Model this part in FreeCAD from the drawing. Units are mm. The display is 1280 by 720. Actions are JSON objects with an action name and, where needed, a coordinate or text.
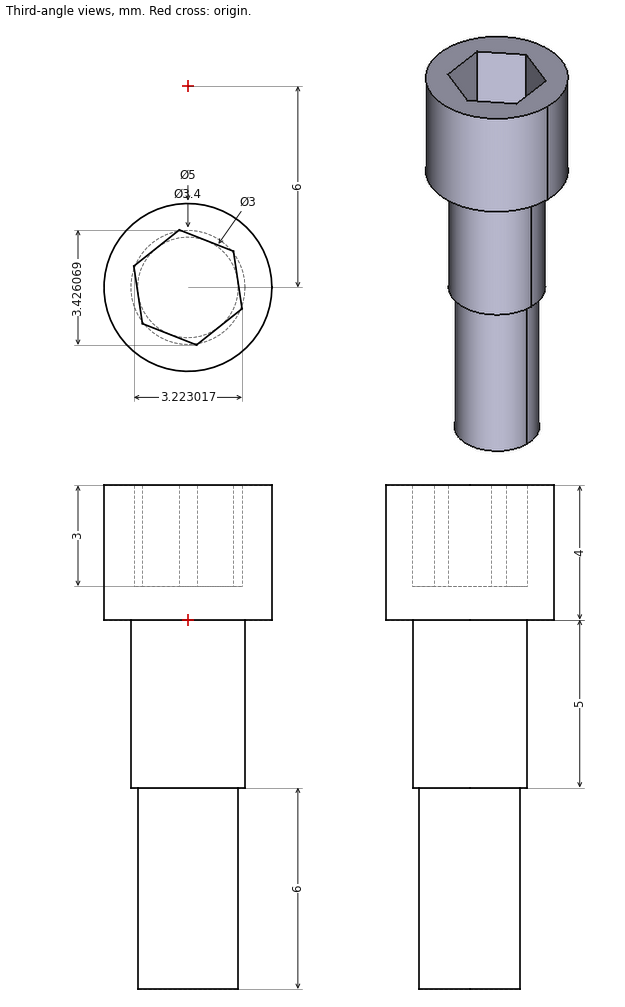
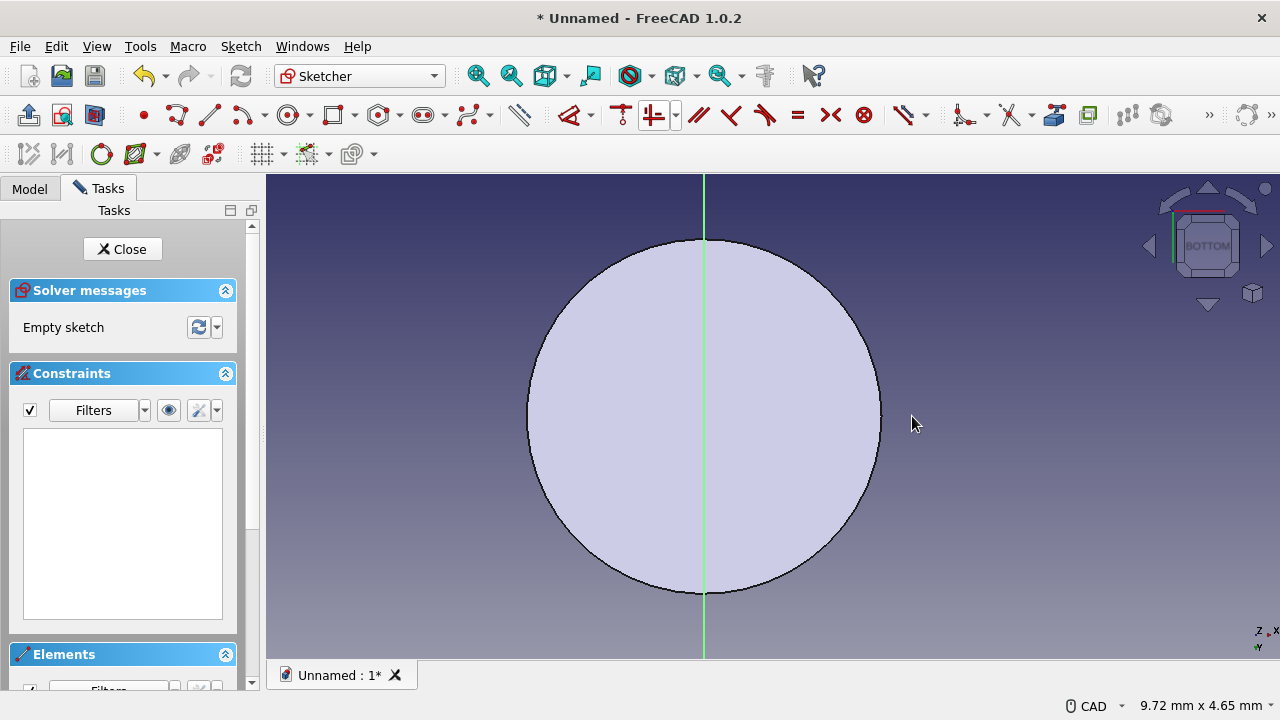
{"action": "key", "text": "g c"}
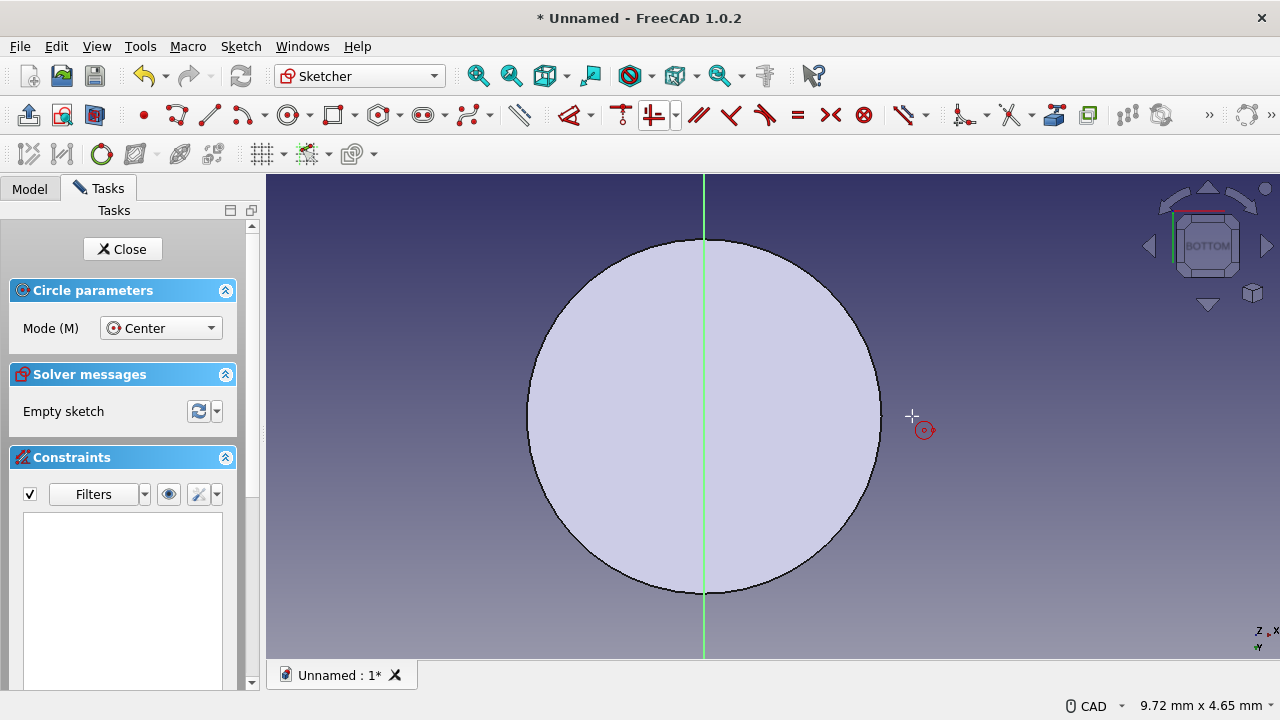
{"action": "left_click", "coordinate": [704, 416]}
{"action": "left_click", "coordinate": [815, 306]}
{"action": "key", "text": "Escape"}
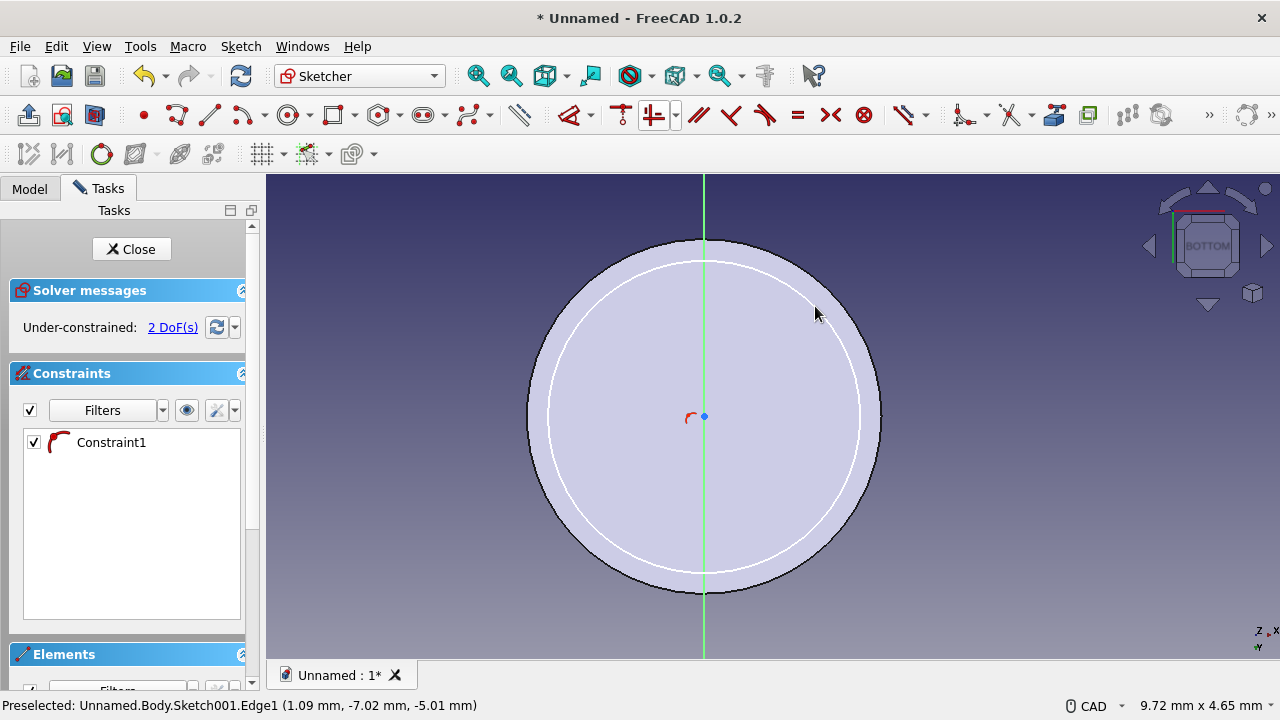
{"action": "left_click", "coordinate": [568, 116]}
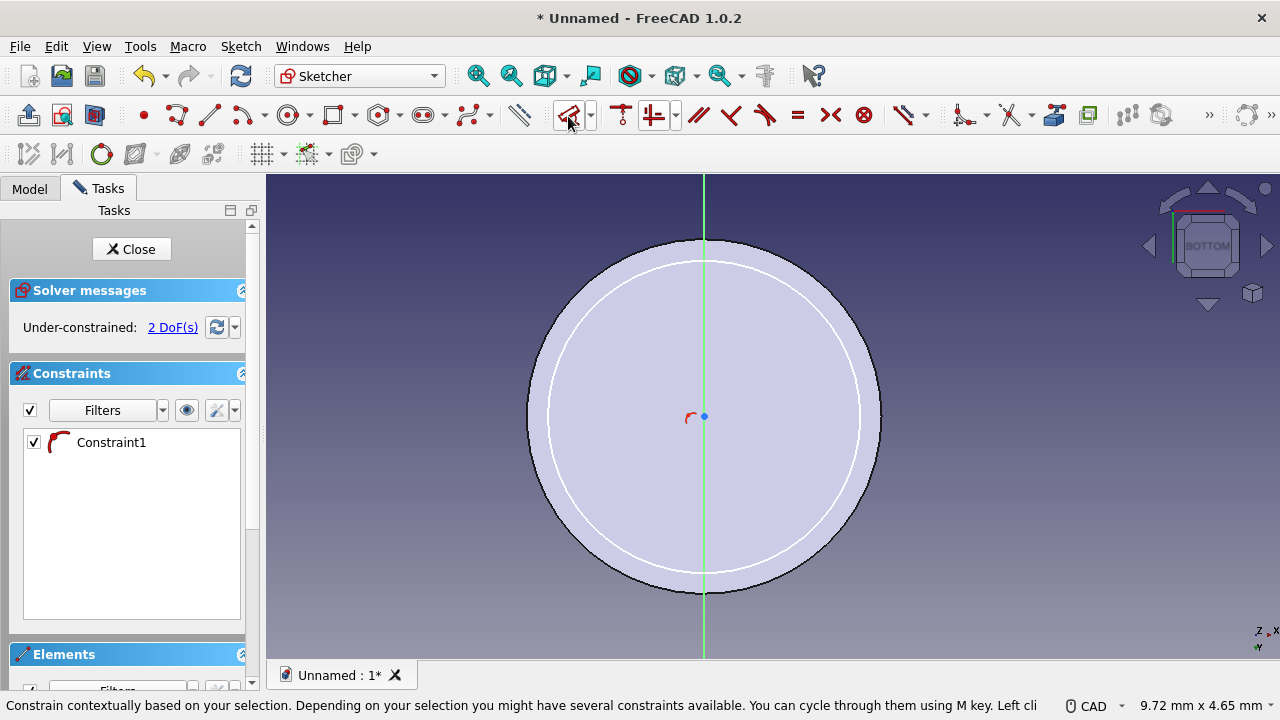
{"action": "left_click", "coordinate": [814, 306]}
{"action": "left_click", "coordinate": [837, 283]}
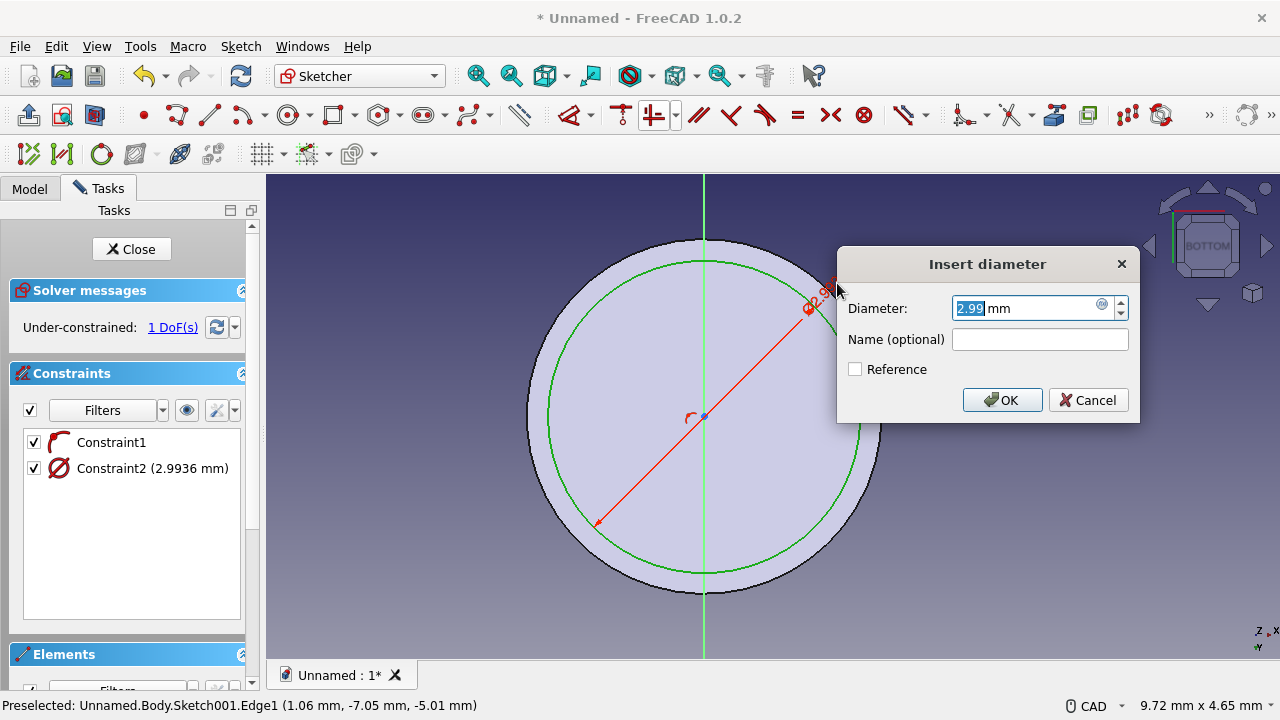
{"action": "type", "text": "3"}
{"action": "key", "text": "Return"}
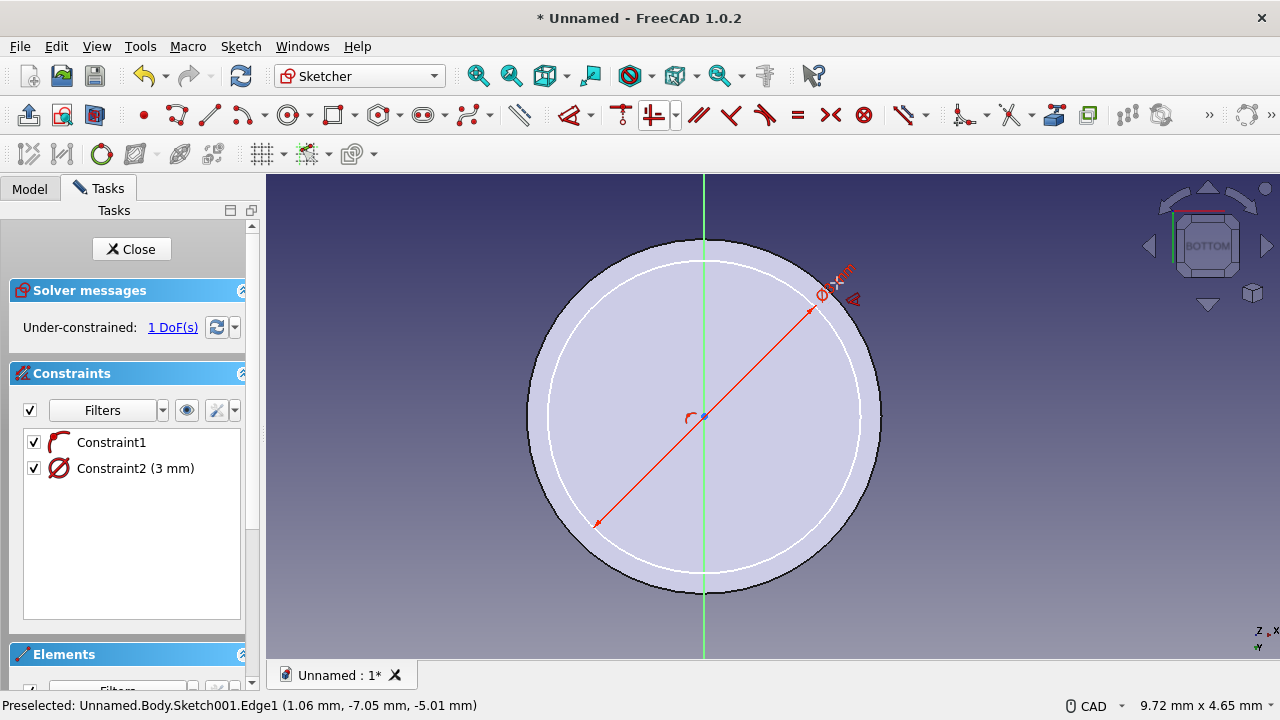
{"action": "scroll", "coordinate": [704, 417], "scroll_direction": "up", "scroll_amount": 4}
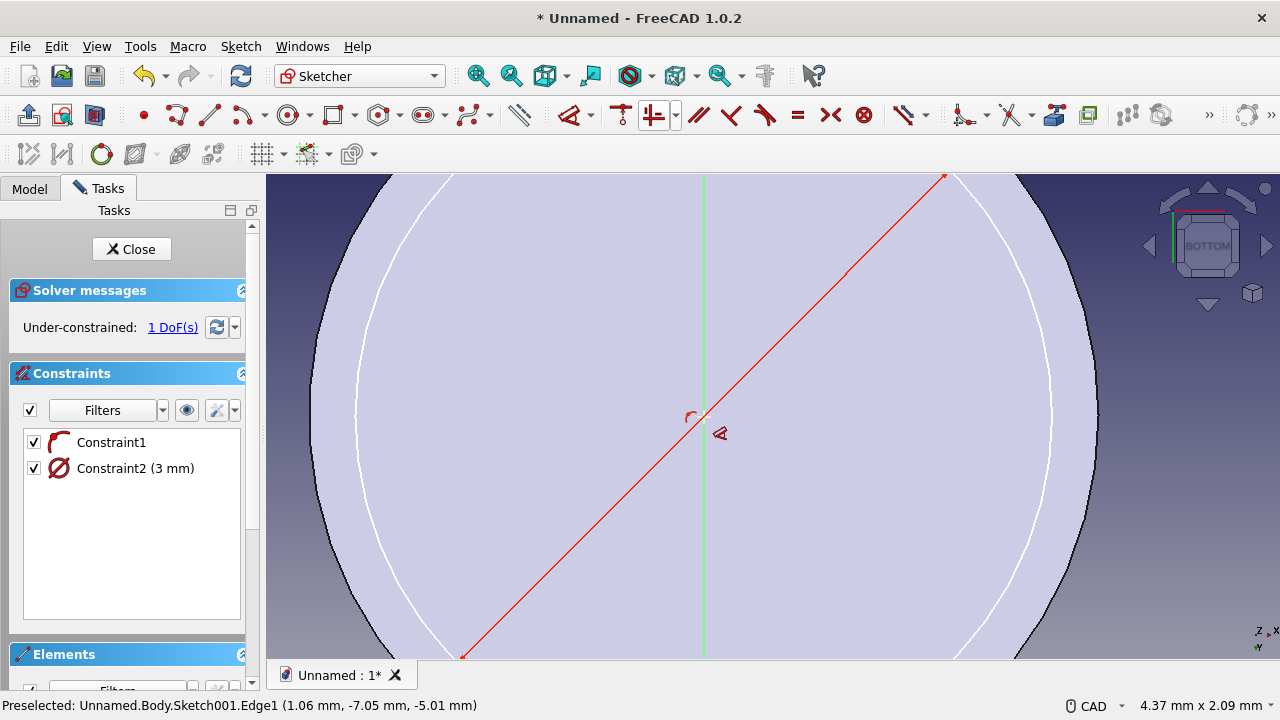
{"action": "left_click", "coordinate": [704, 416]}
{"action": "left_click", "coordinate": [738, 524]}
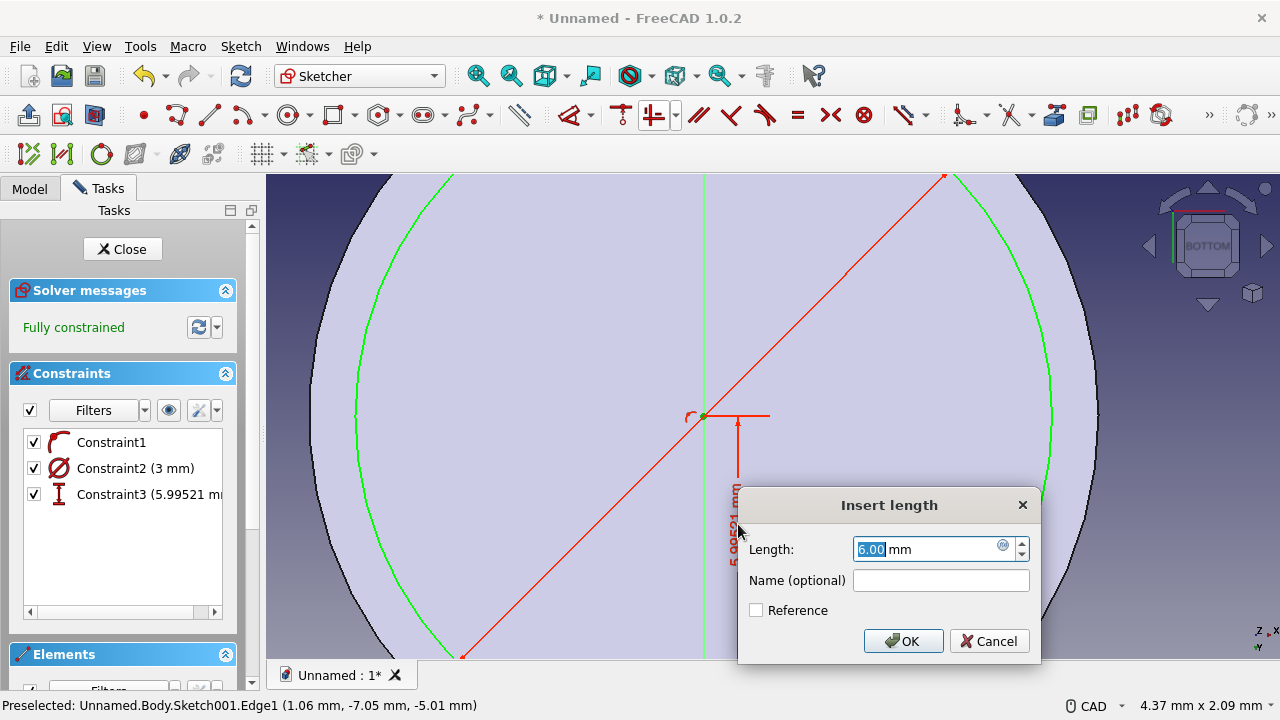
{"action": "type", "text": "6"}
{"action": "key", "text": "Return"}
{"action": "key", "text": "Escape"}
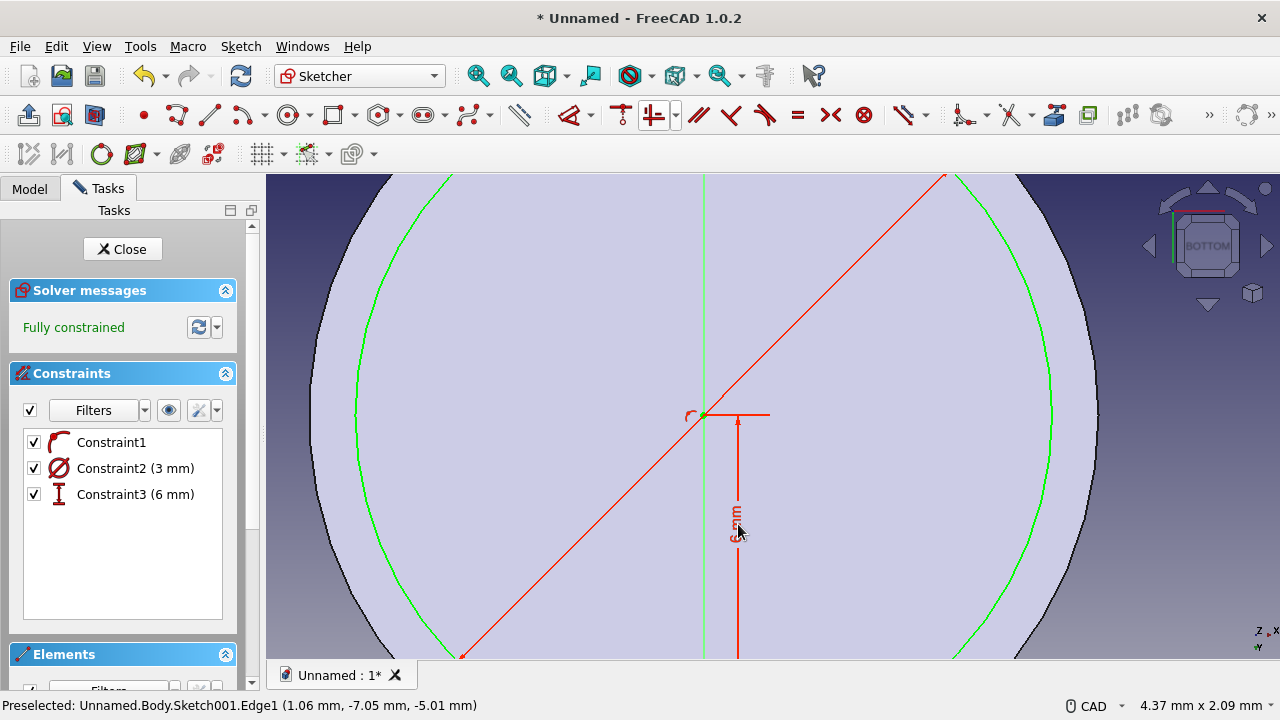
{"action": "left_click", "coordinate": [123, 249]}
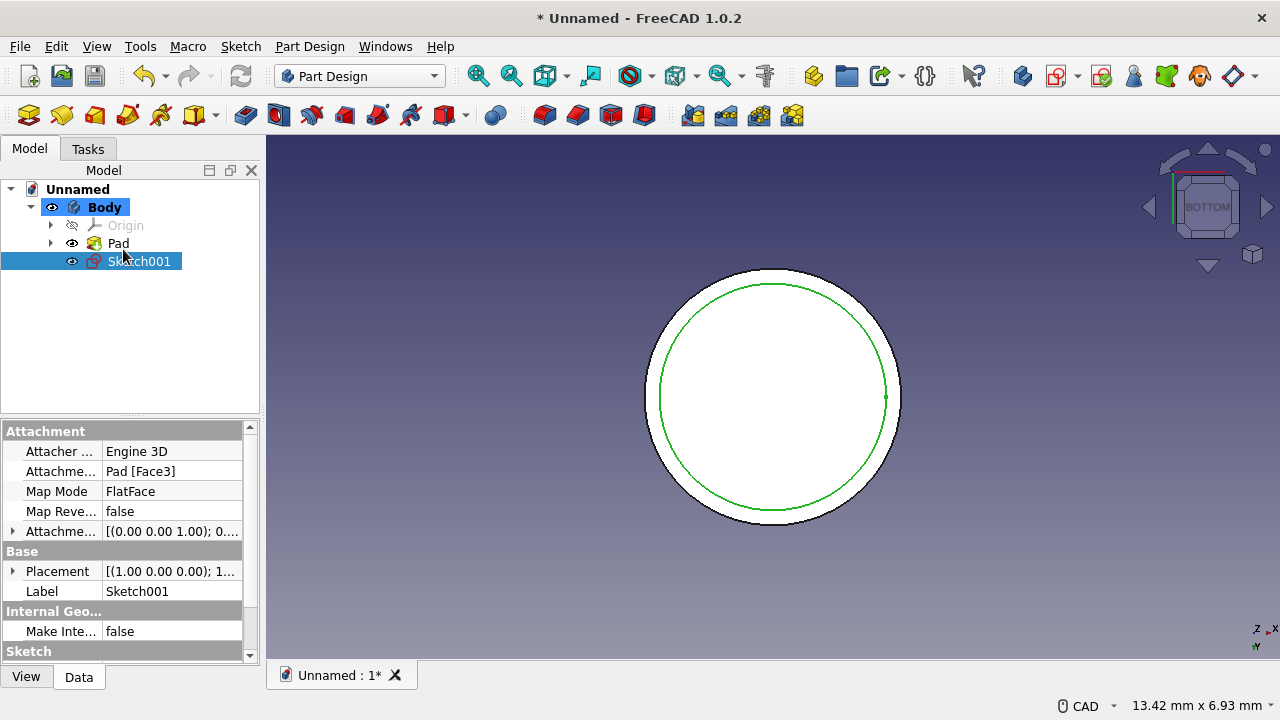
{"action": "left_click", "coordinate": [29, 116]}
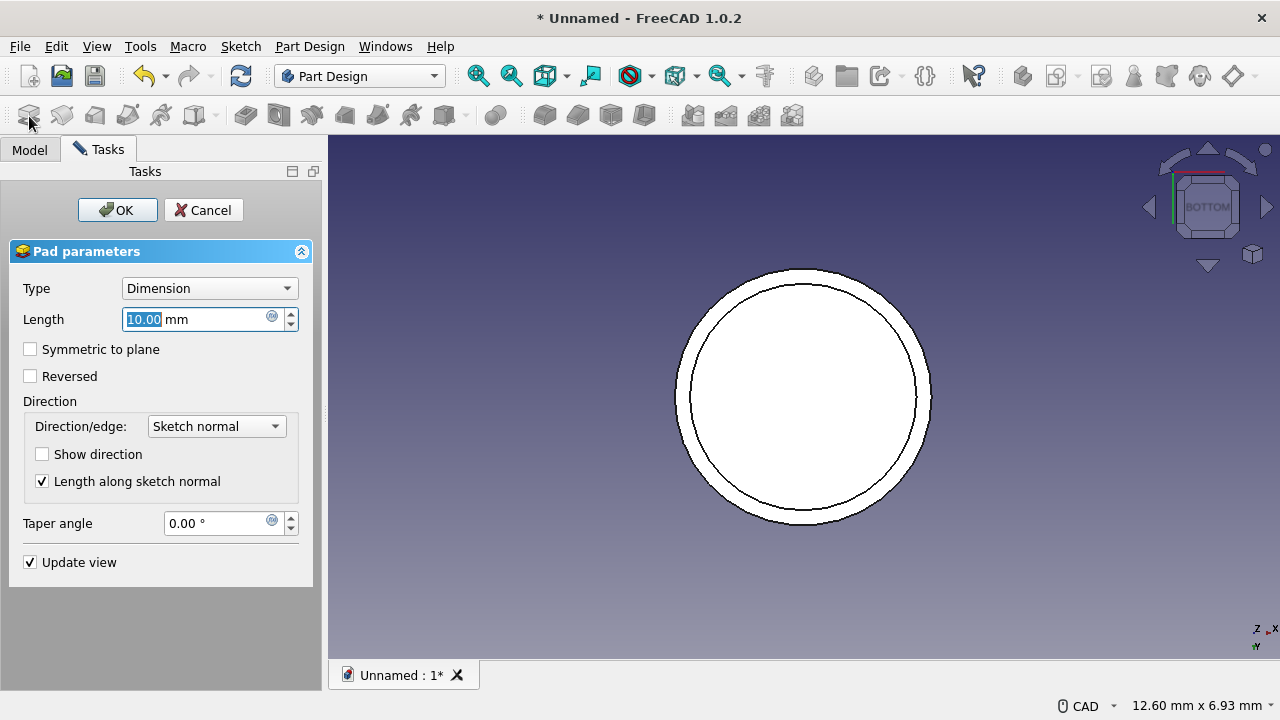
{"action": "type", "text": "6"}
{"action": "key", "text": "Tab"}